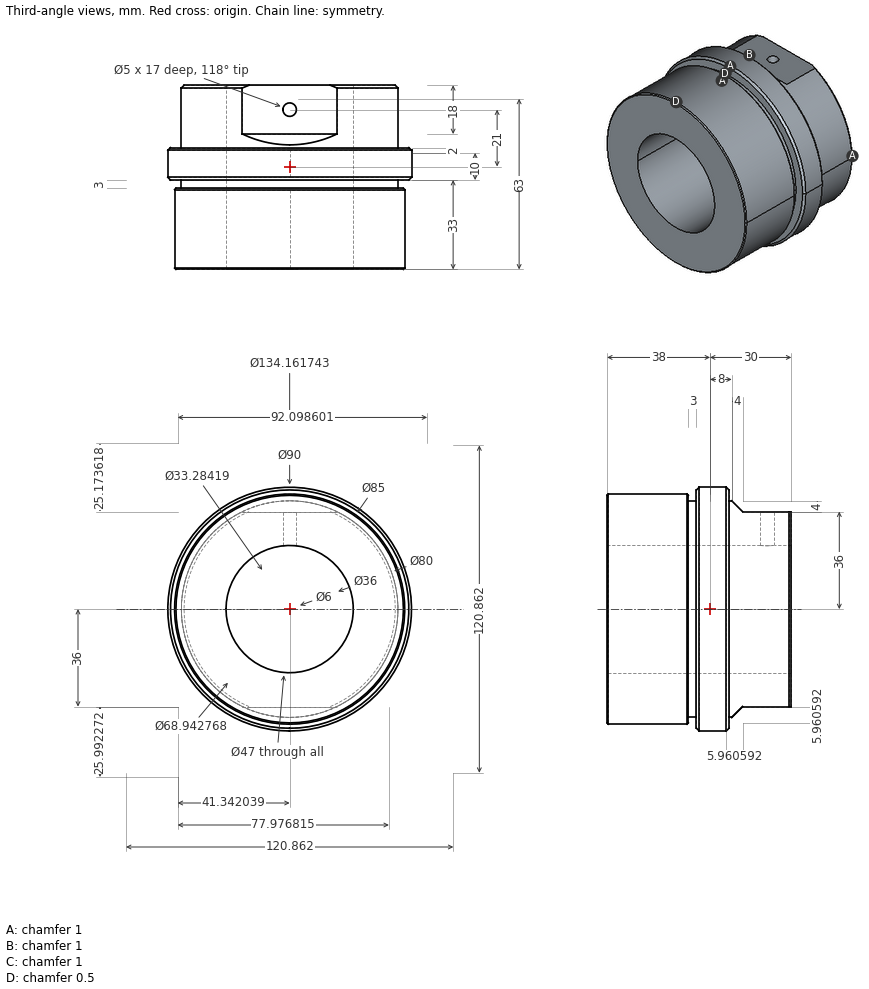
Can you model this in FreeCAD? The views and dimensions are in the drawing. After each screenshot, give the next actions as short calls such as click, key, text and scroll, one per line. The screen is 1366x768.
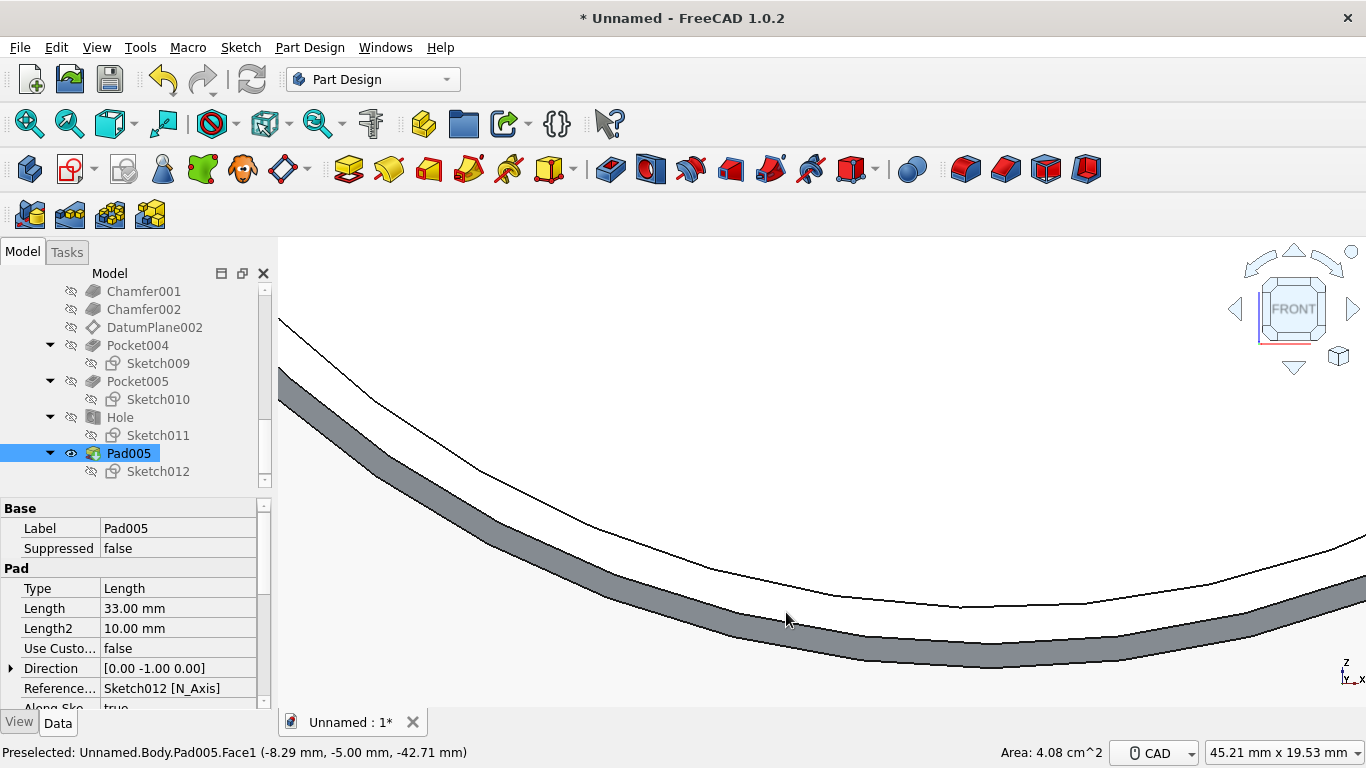
click(70, 170)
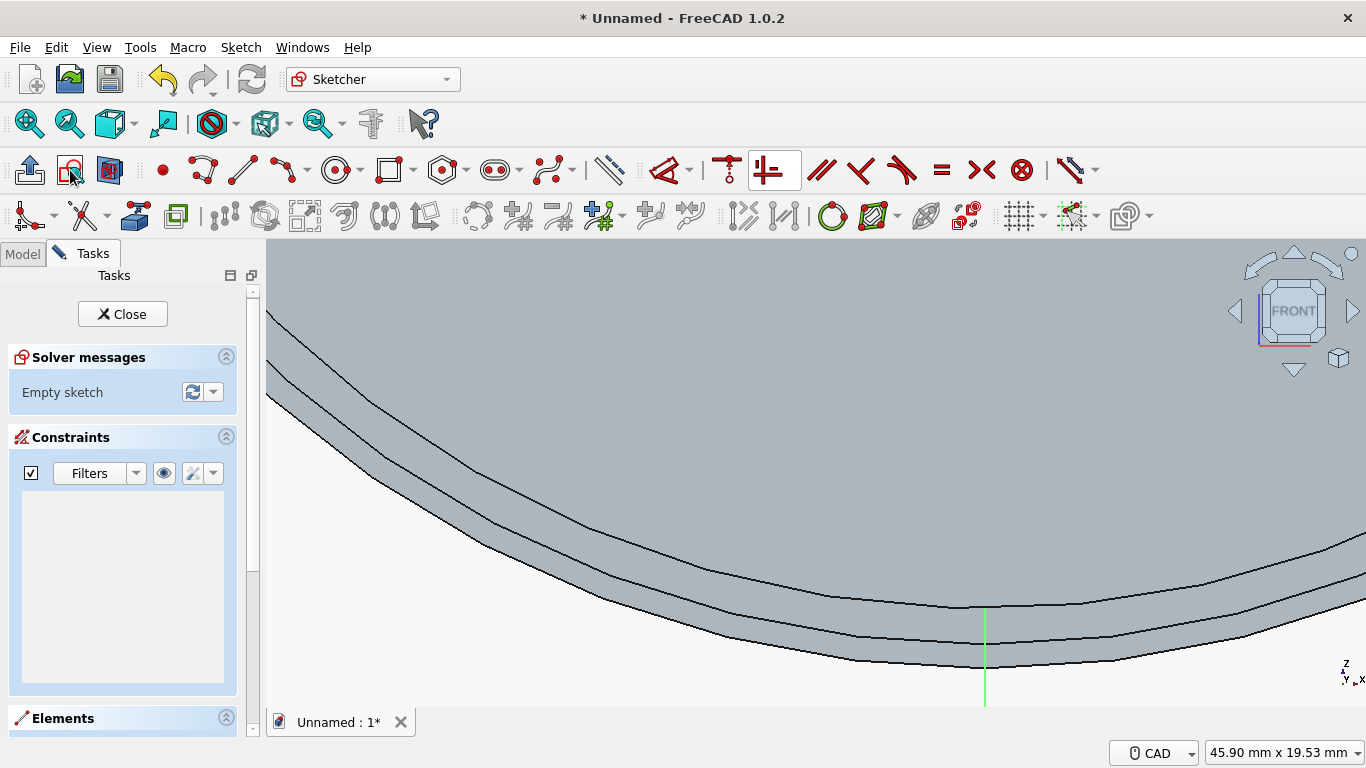
scroll(718, 583, down, 11)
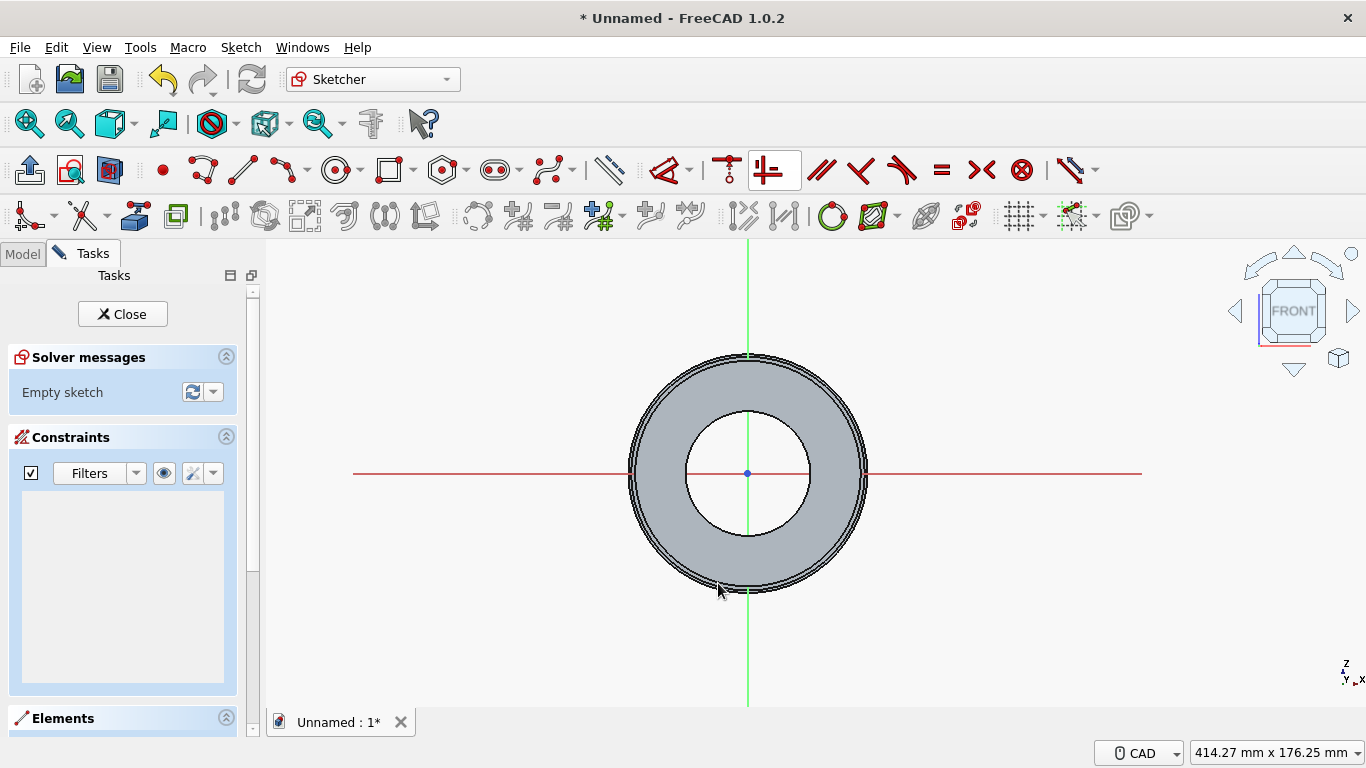
key(g)
key(v)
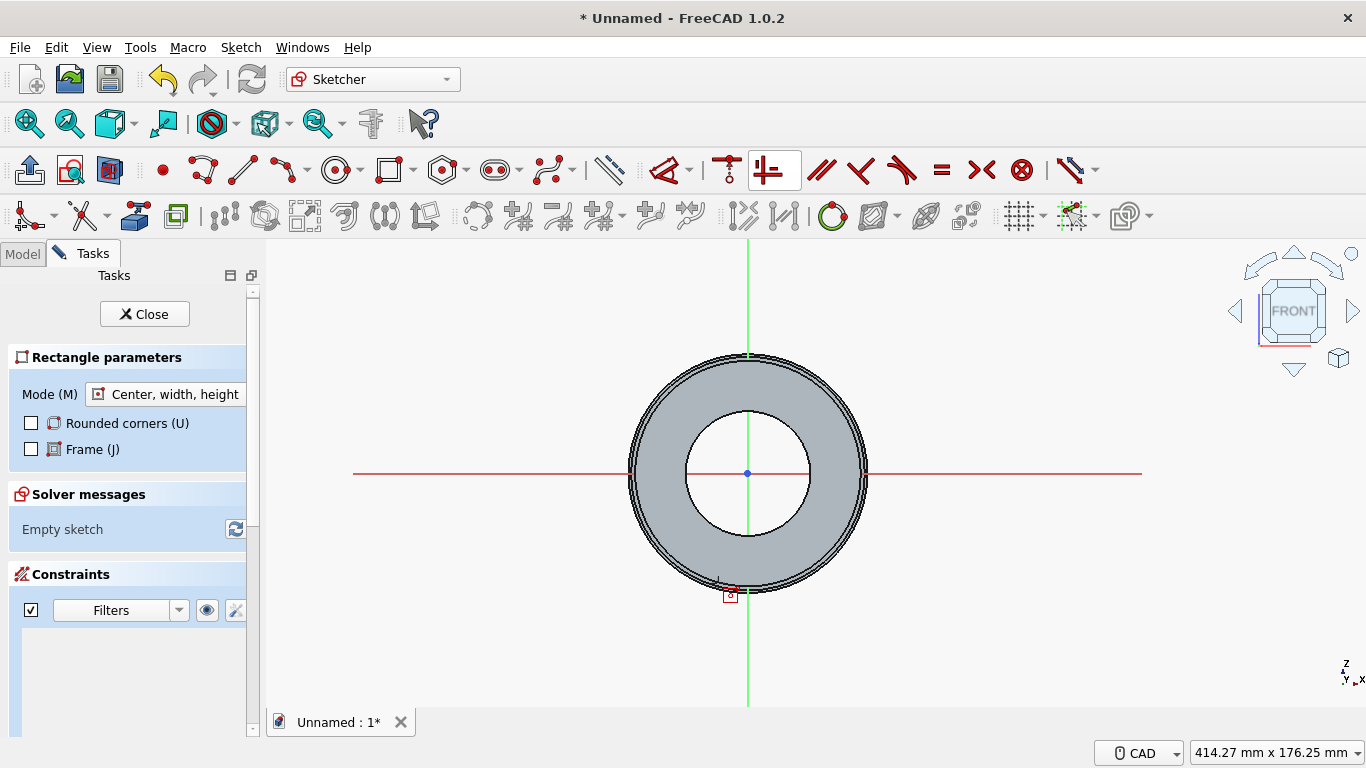
click(748, 474)
click(908, 313)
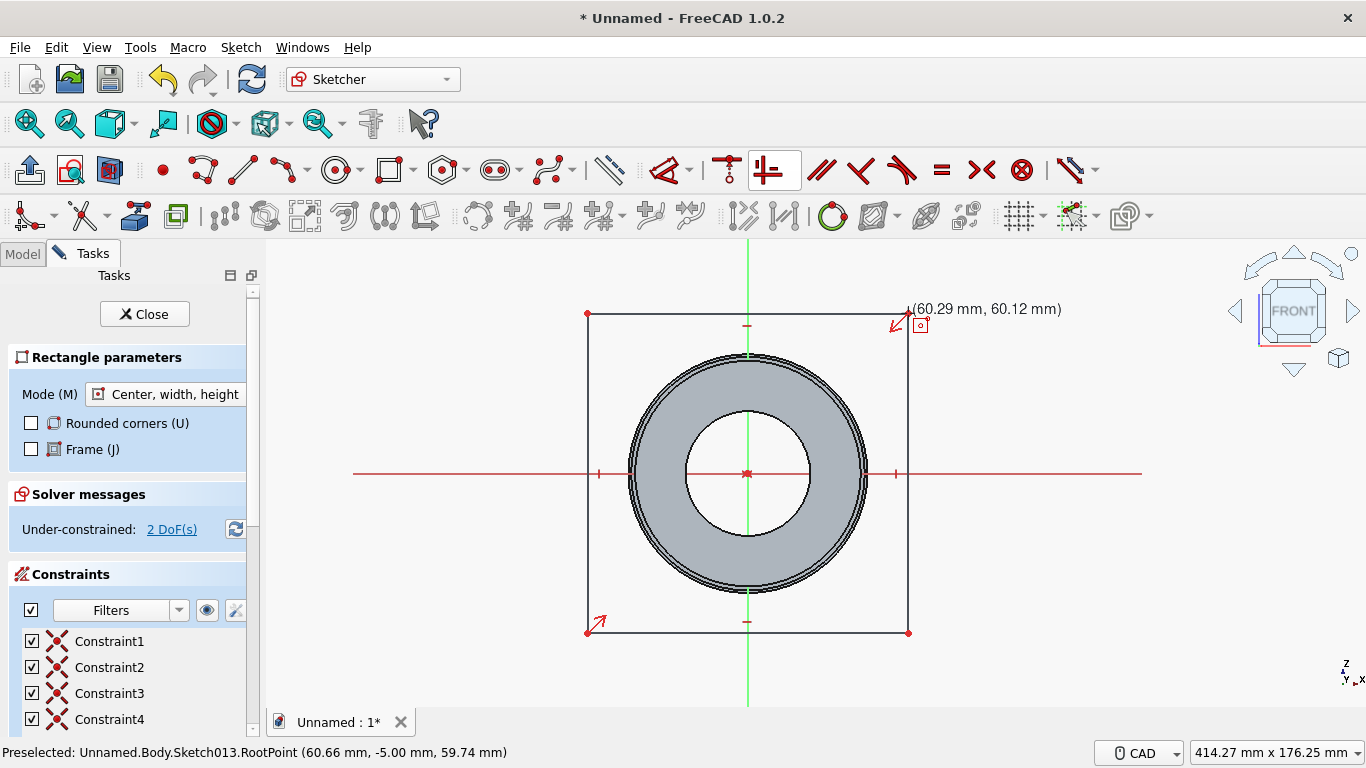
click(336, 170)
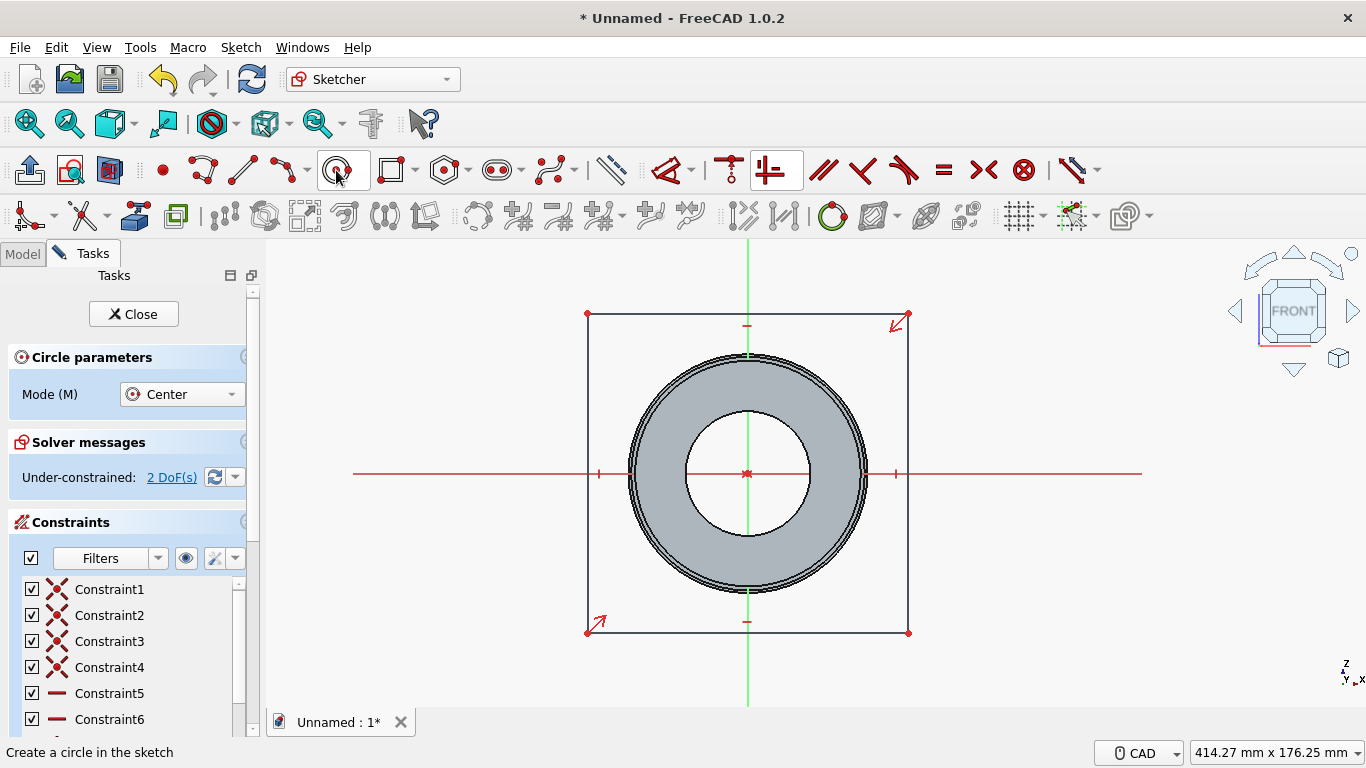
click(748, 474)
click(823, 399)
key(Escape)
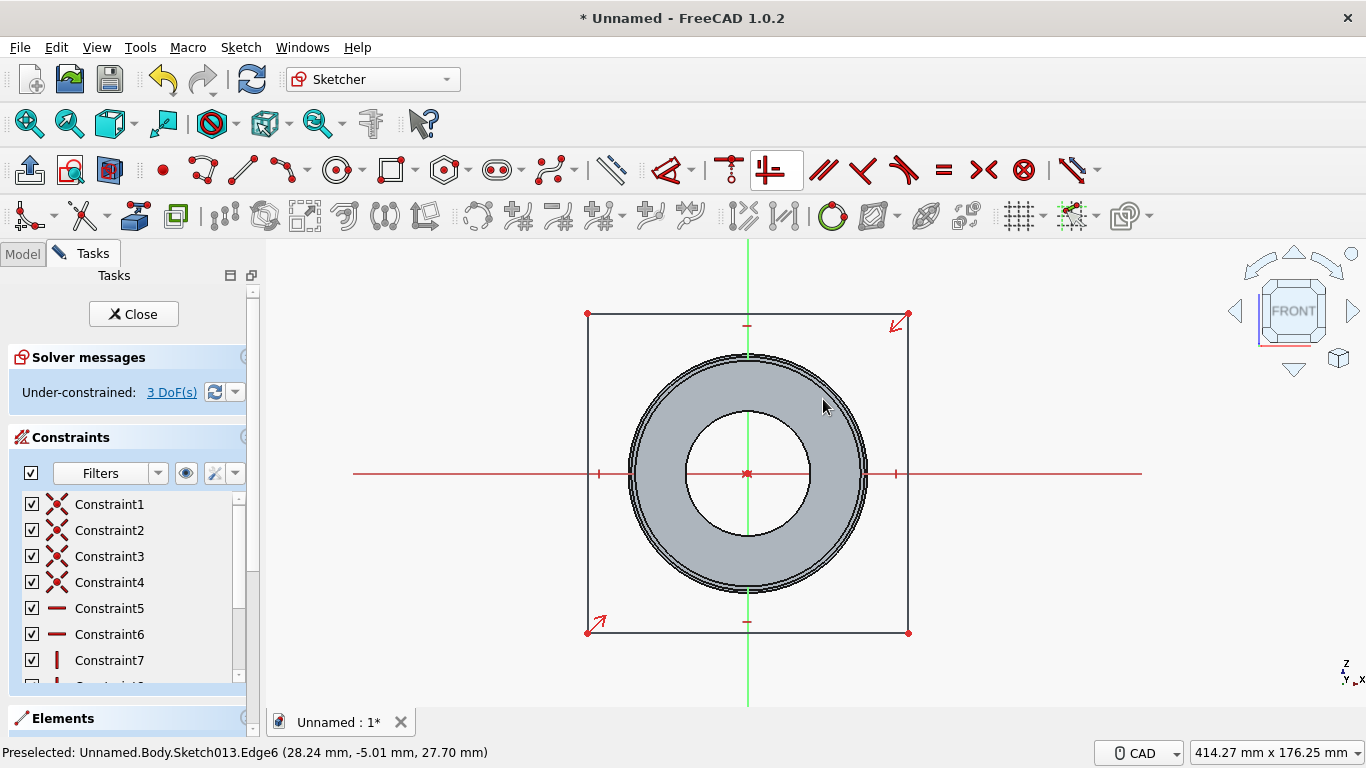
click(666, 170)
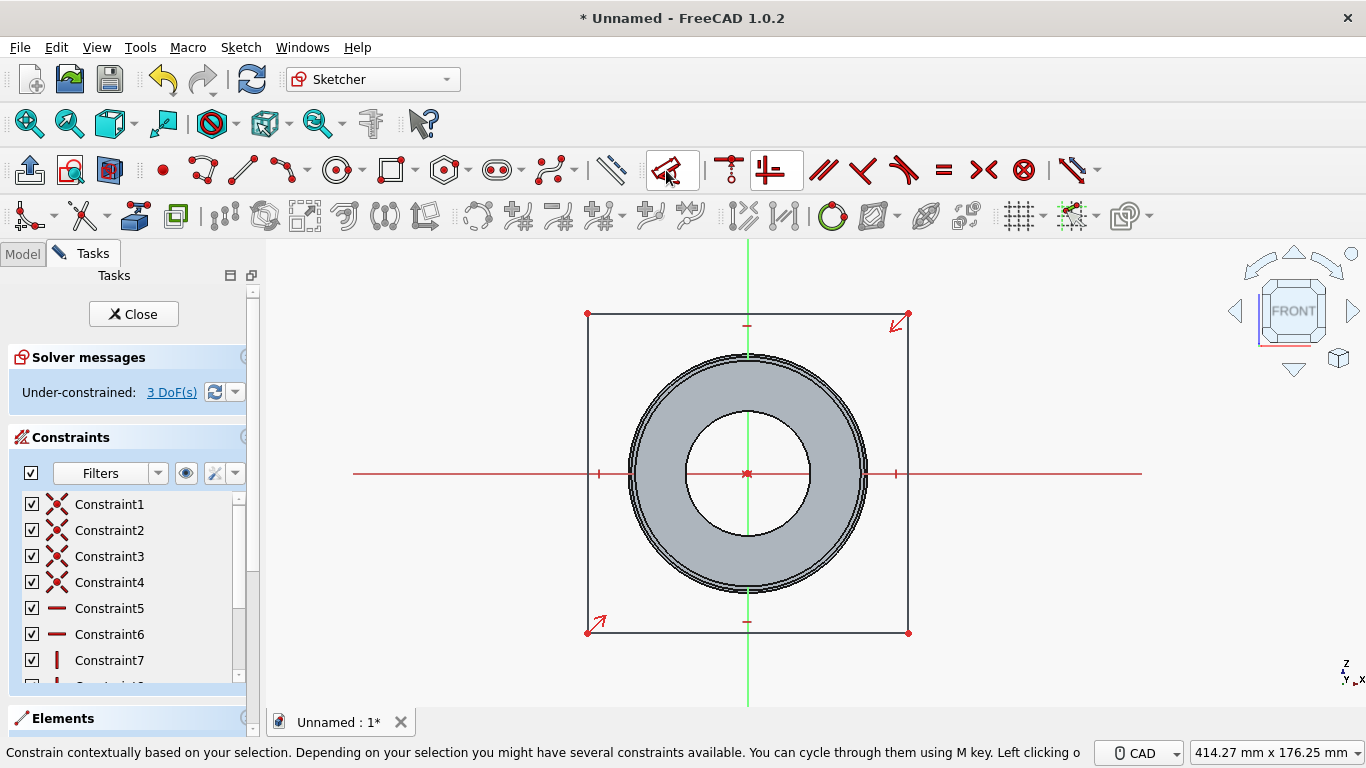
click(822, 399)
click(845, 376)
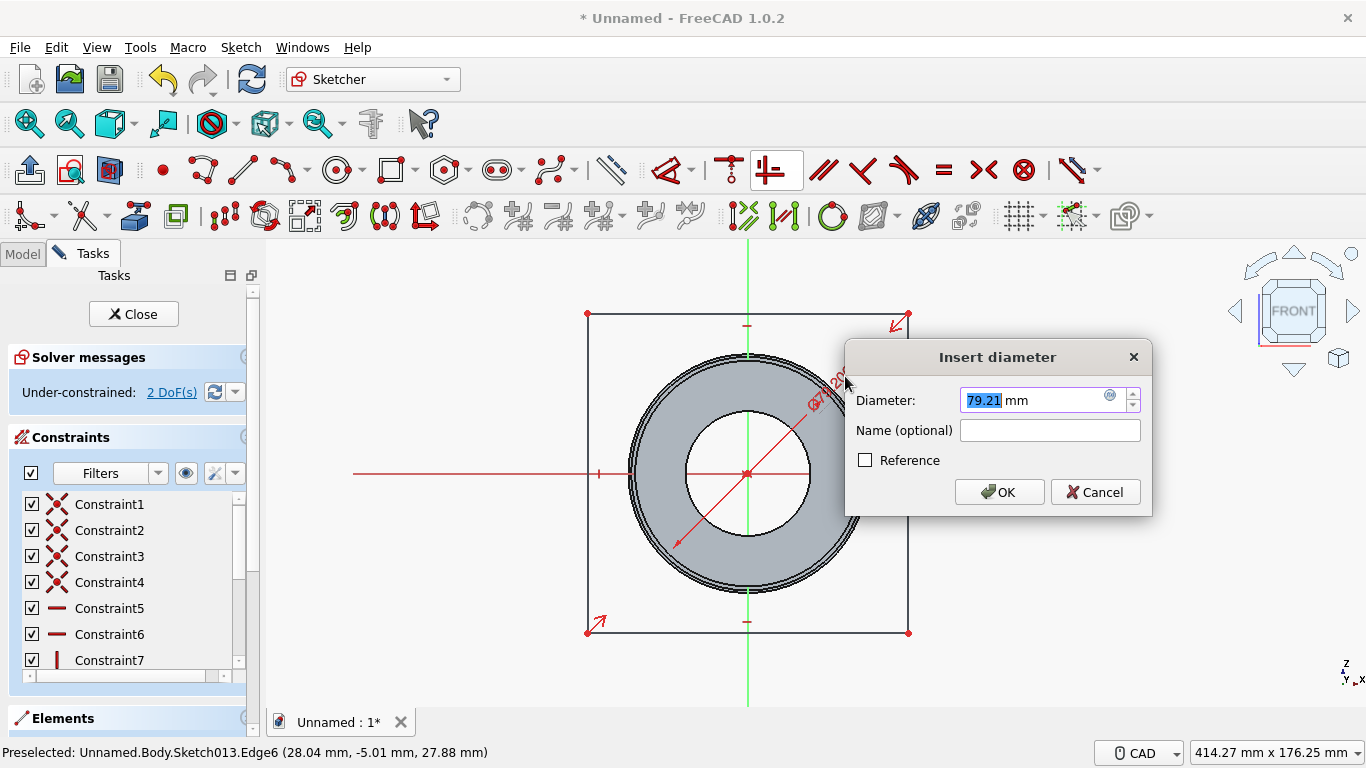
text(80)
key(Return)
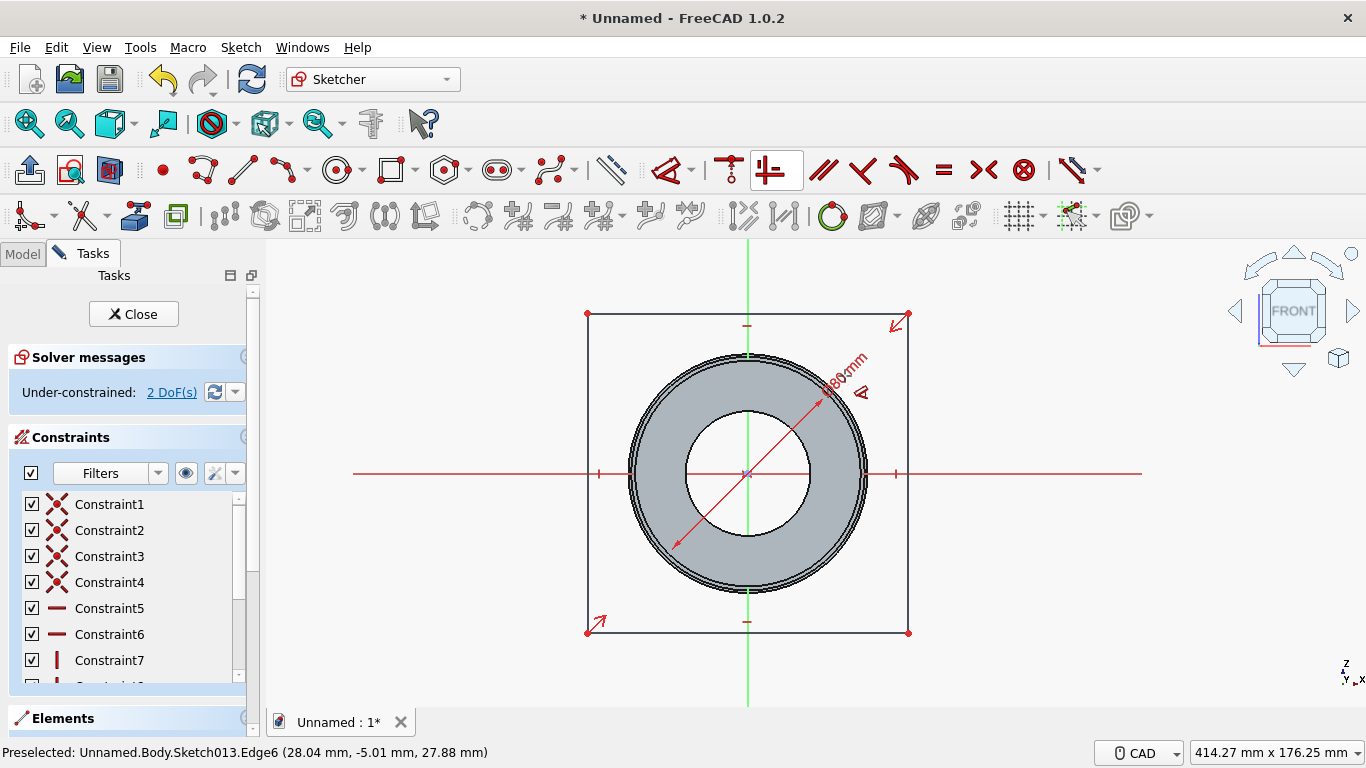
click(684, 633)
click(674, 667)